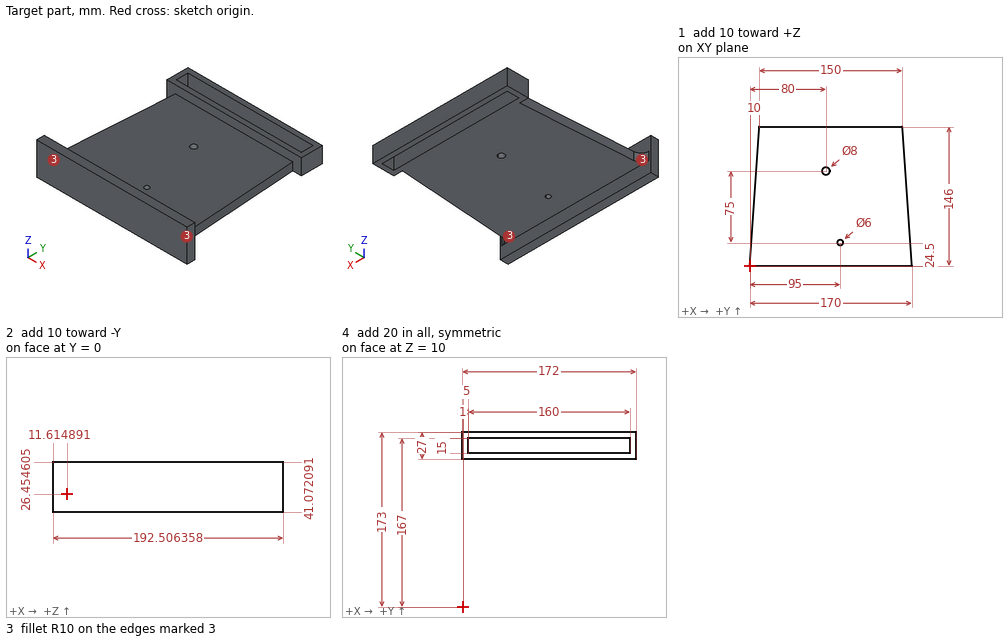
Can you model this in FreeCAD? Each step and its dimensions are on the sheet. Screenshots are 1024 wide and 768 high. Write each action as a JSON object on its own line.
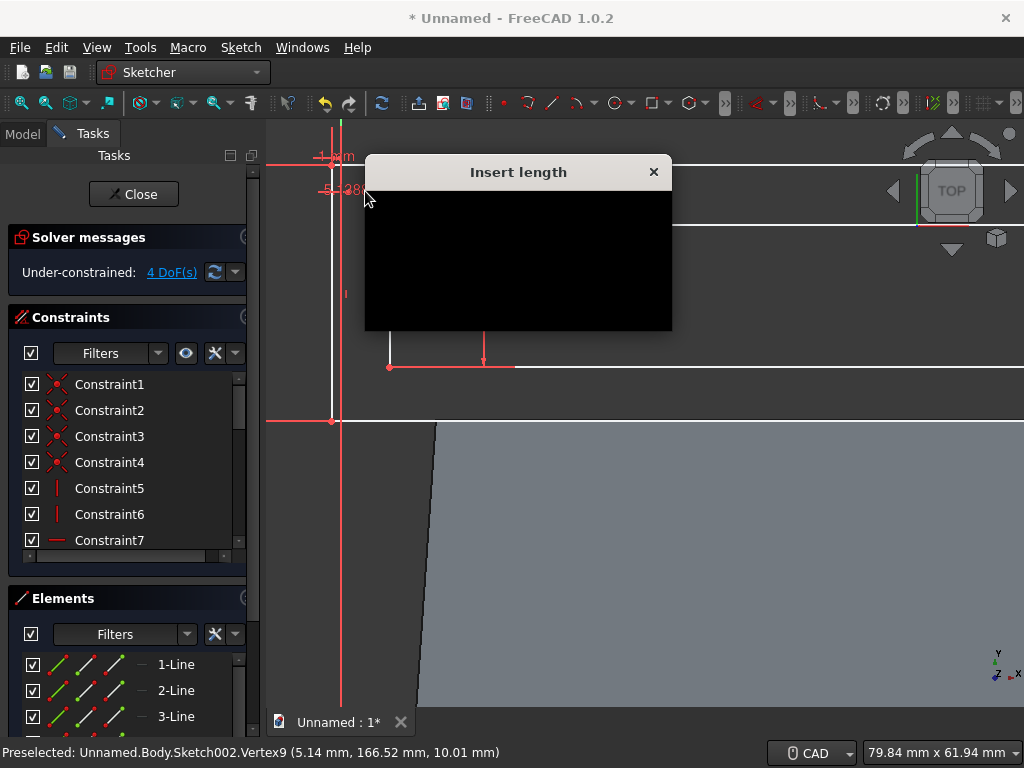
{"action": "type", "text": "5"}
{"action": "key", "text": "Return"}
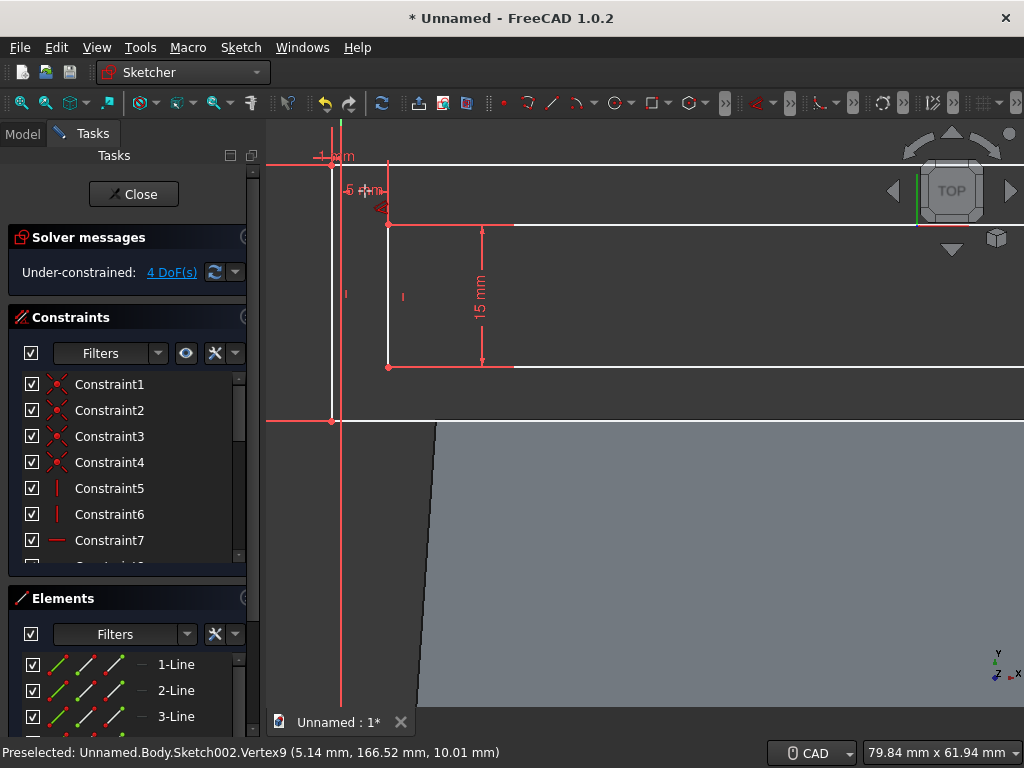
{"action": "scroll", "coordinate": [389, 226], "scroll_direction": "down", "scroll_amount": 7}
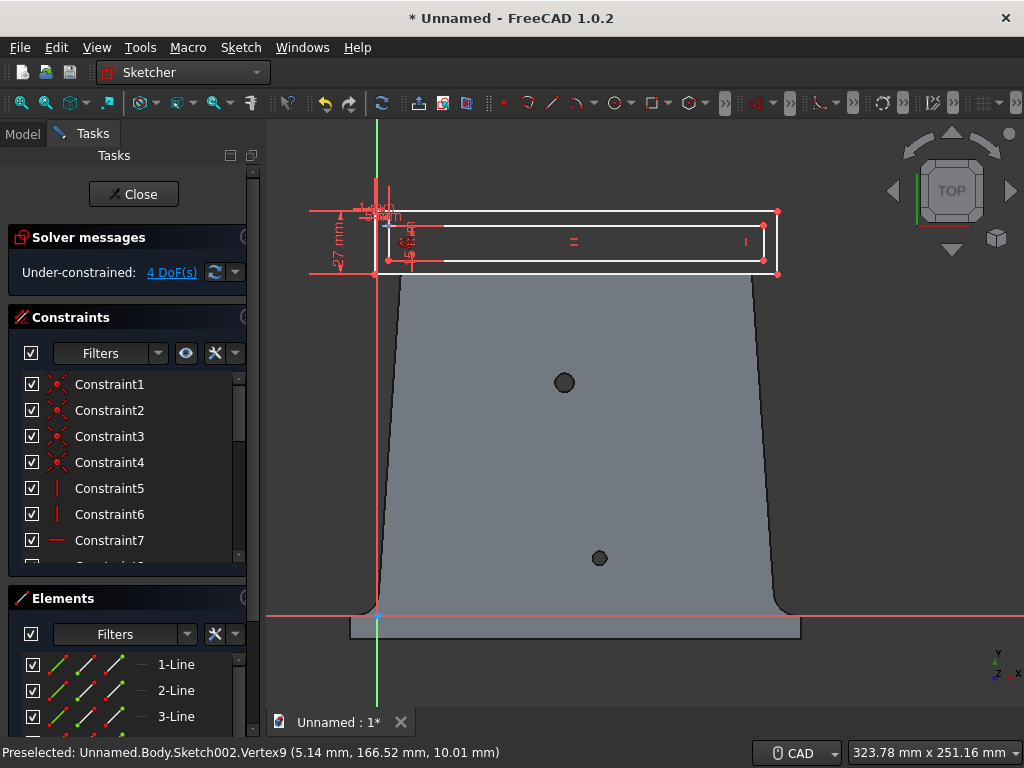
{"action": "left_click", "coordinate": [496, 274]}
{"action": "left_click", "coordinate": [576, 240]}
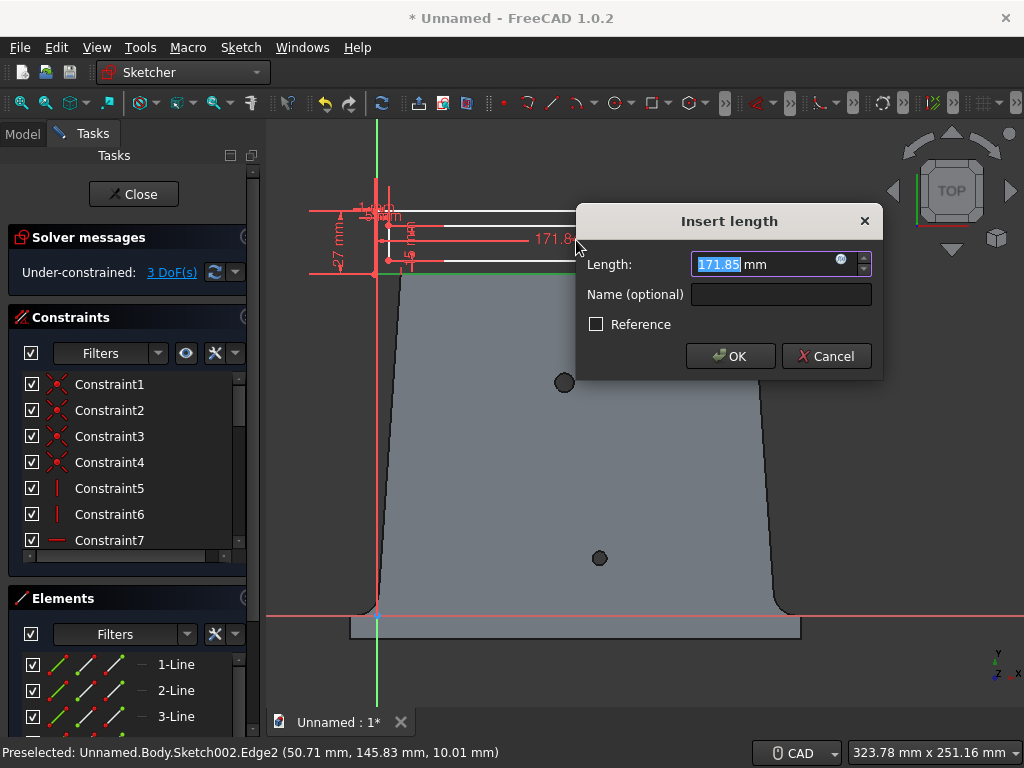
{"action": "type", "text": "172"}
{"action": "key", "text": "Return"}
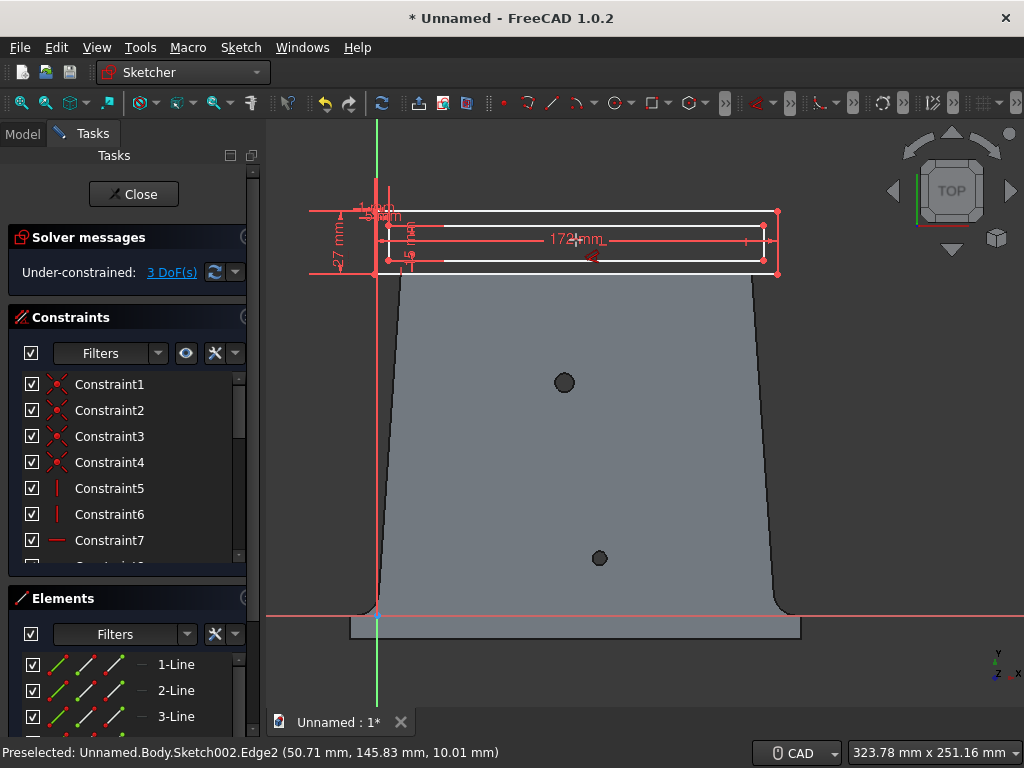
{"action": "left_click", "coordinate": [501, 261]}
{"action": "left_click", "coordinate": [576, 295]}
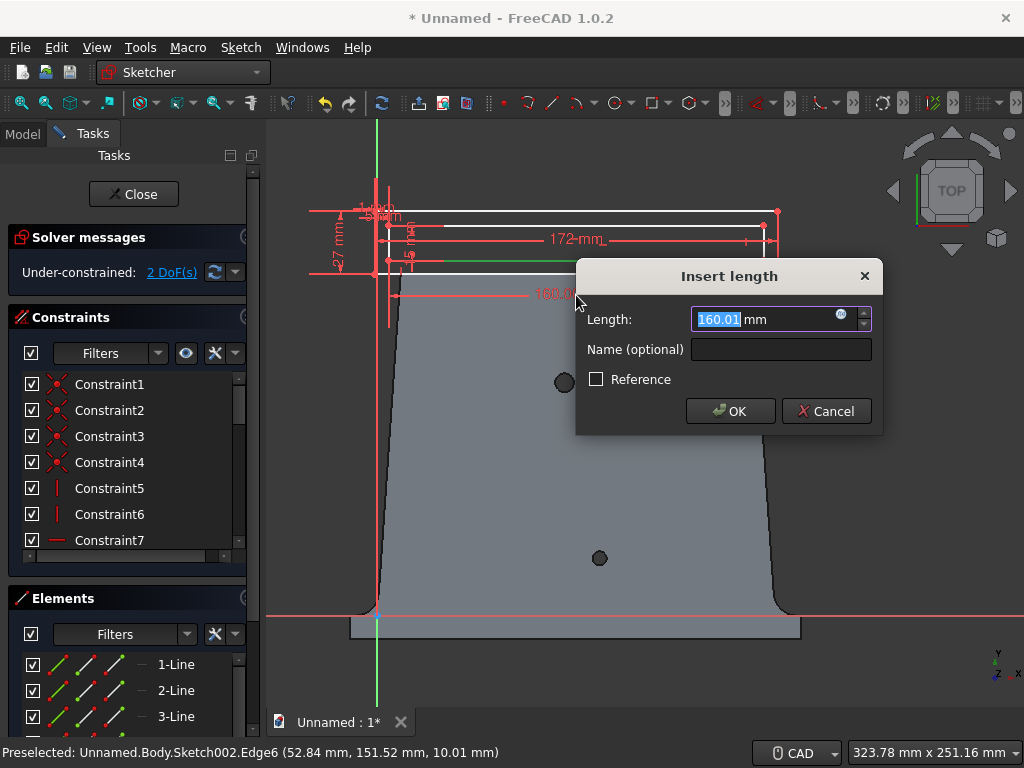
{"action": "type", "text": "160"}
{"action": "key", "text": "Return"}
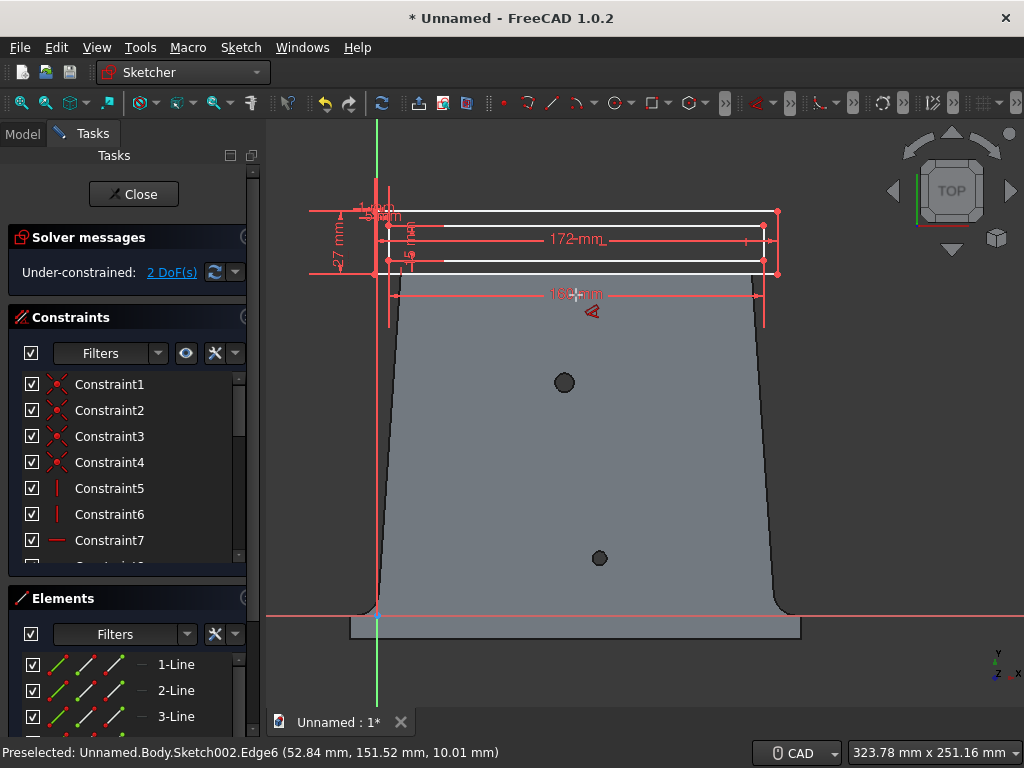
{"action": "left_click", "coordinate": [375, 211]}
{"action": "left_click", "coordinate": [341, 413]}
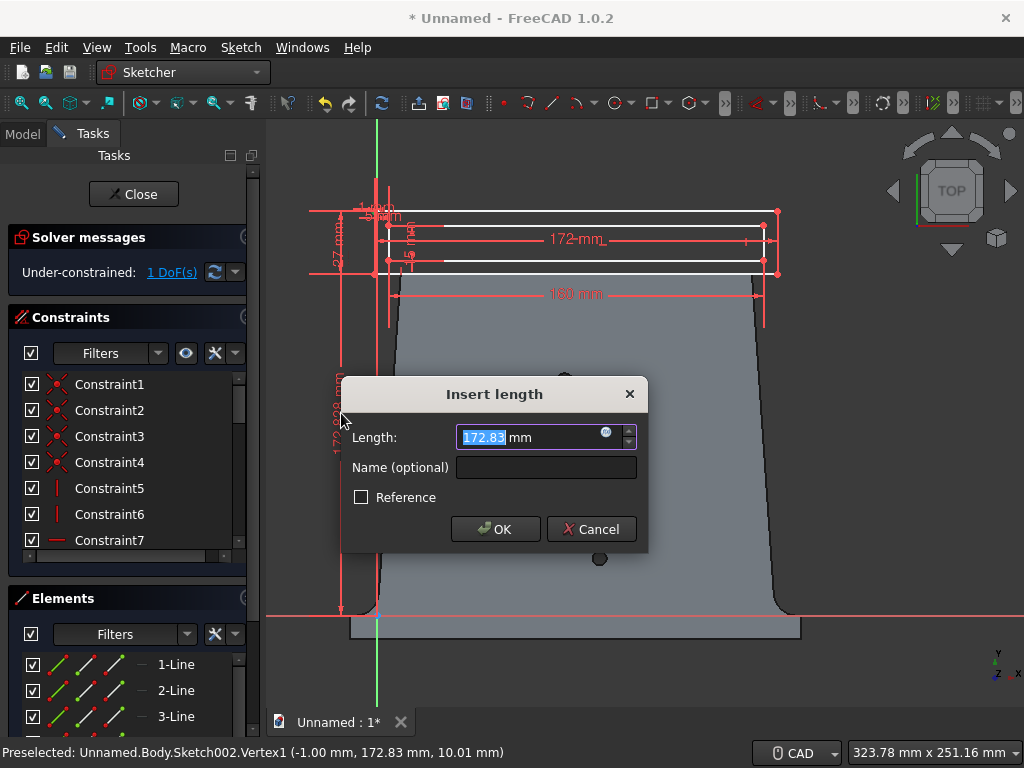
{"action": "type", "text": "173"}
{"action": "key", "text": "Return"}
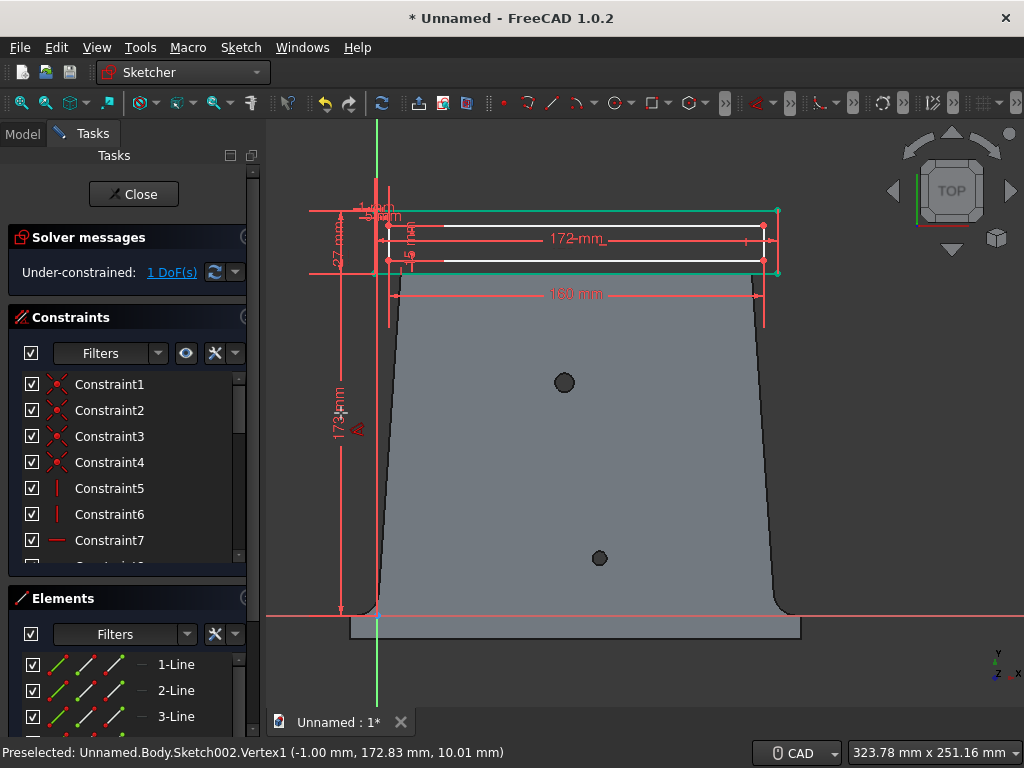
{"action": "left_click", "coordinate": [389, 226]}
{"action": "left_click", "coordinate": [343, 331]}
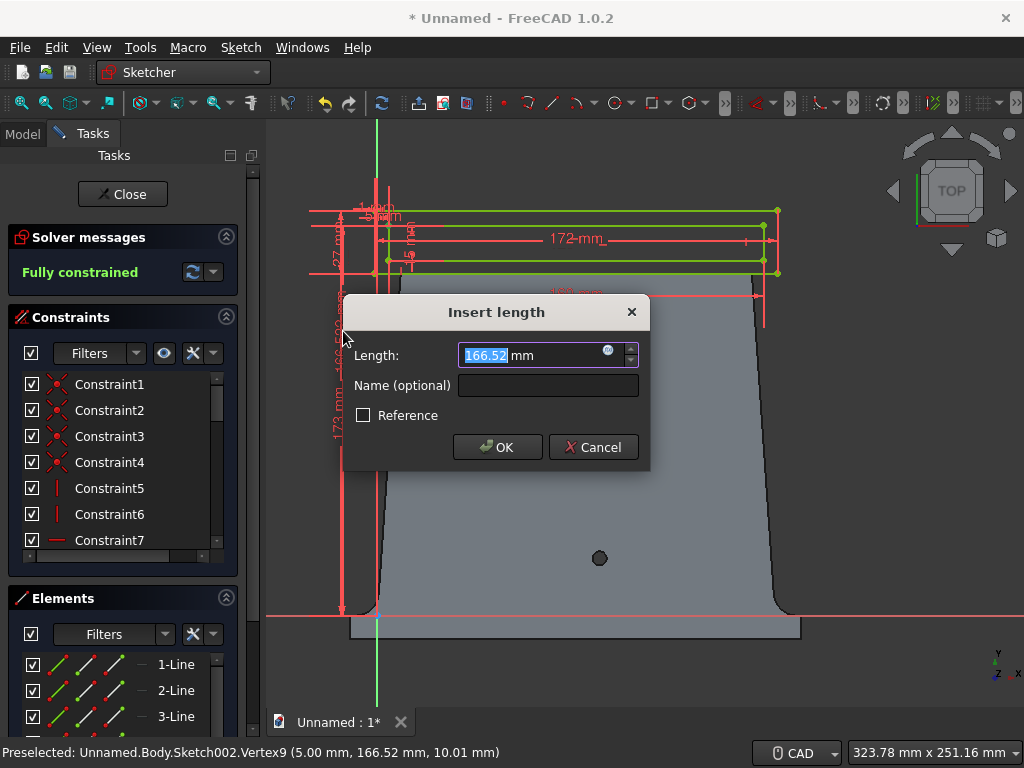
{"action": "type", "text": "167"}
{"action": "key", "text": "Return"}
{"action": "key", "text": "Escape"}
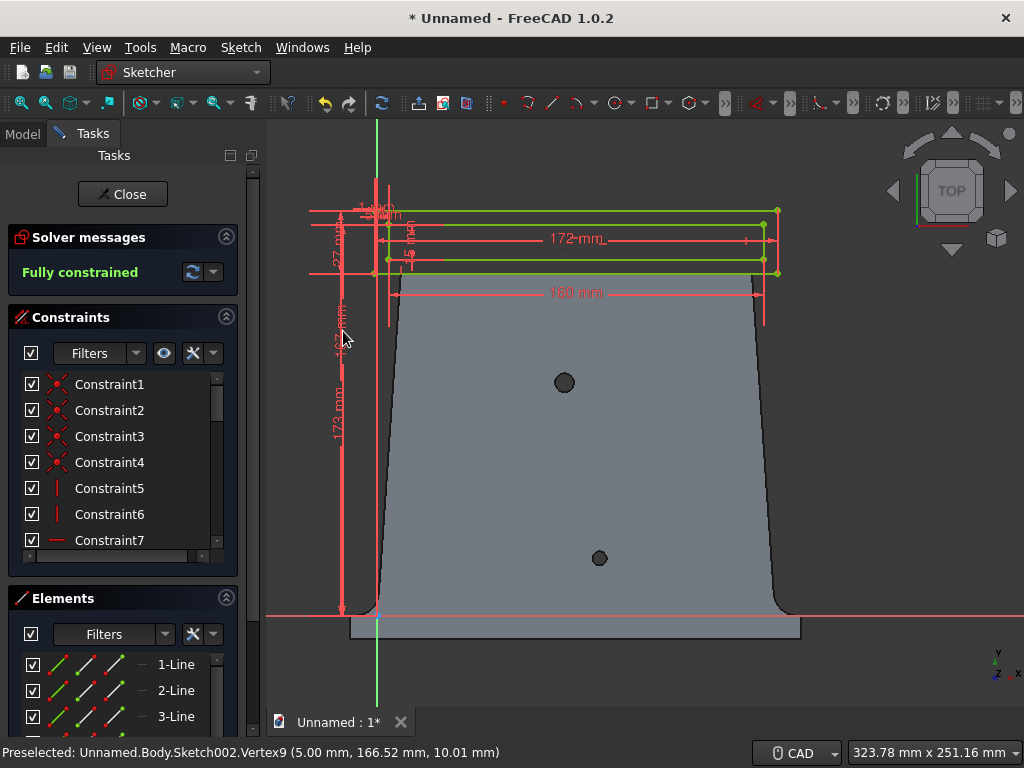
{"action": "left_click", "coordinate": [123, 194]}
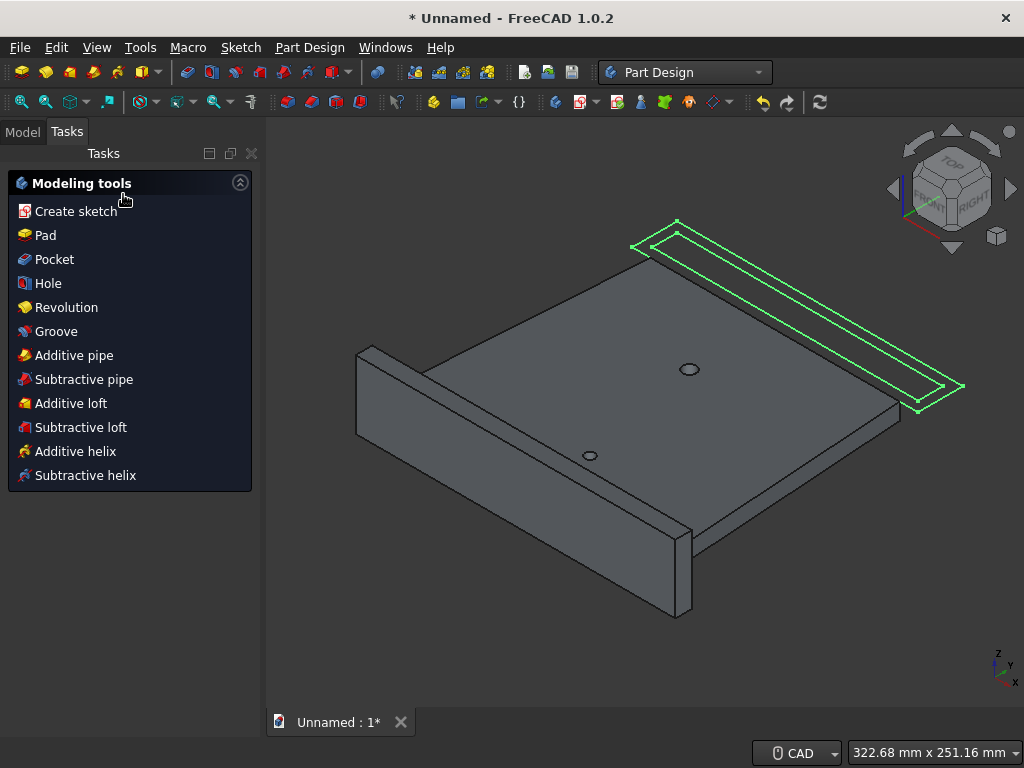
{"action": "left_click", "coordinate": [22, 72]}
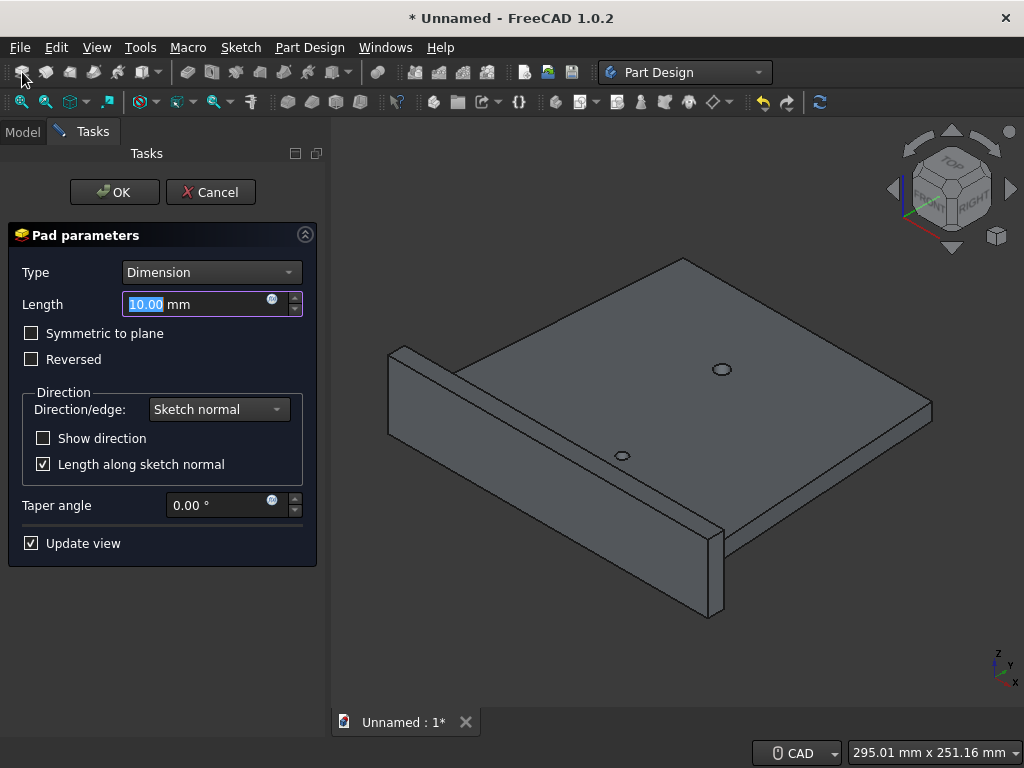
{"action": "type", "text": "20"}
{"action": "key", "text": "Tab"}